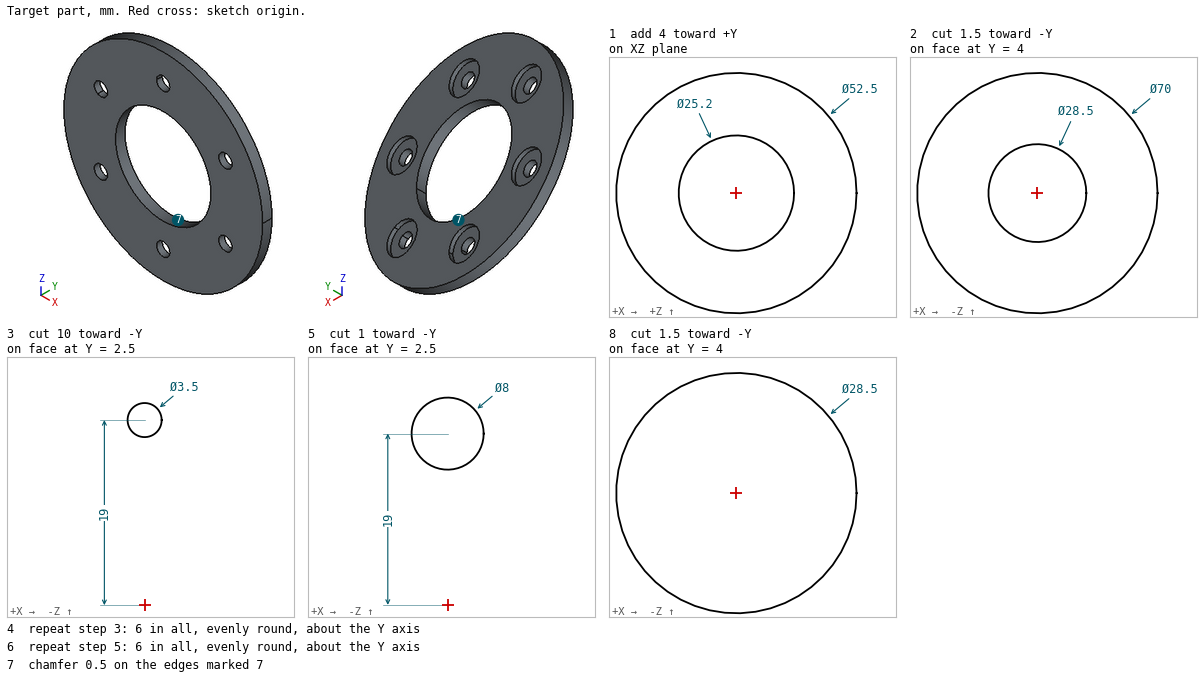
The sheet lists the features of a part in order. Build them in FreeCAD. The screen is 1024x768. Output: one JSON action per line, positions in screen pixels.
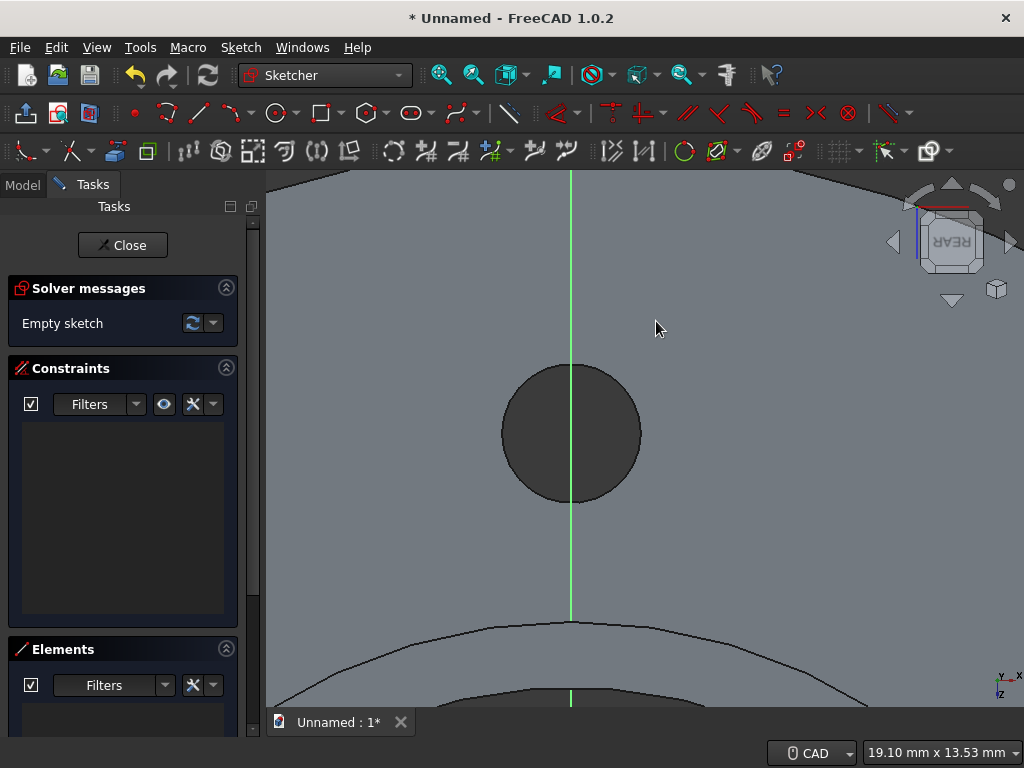
{"action": "left_click", "coordinate": [276, 114]}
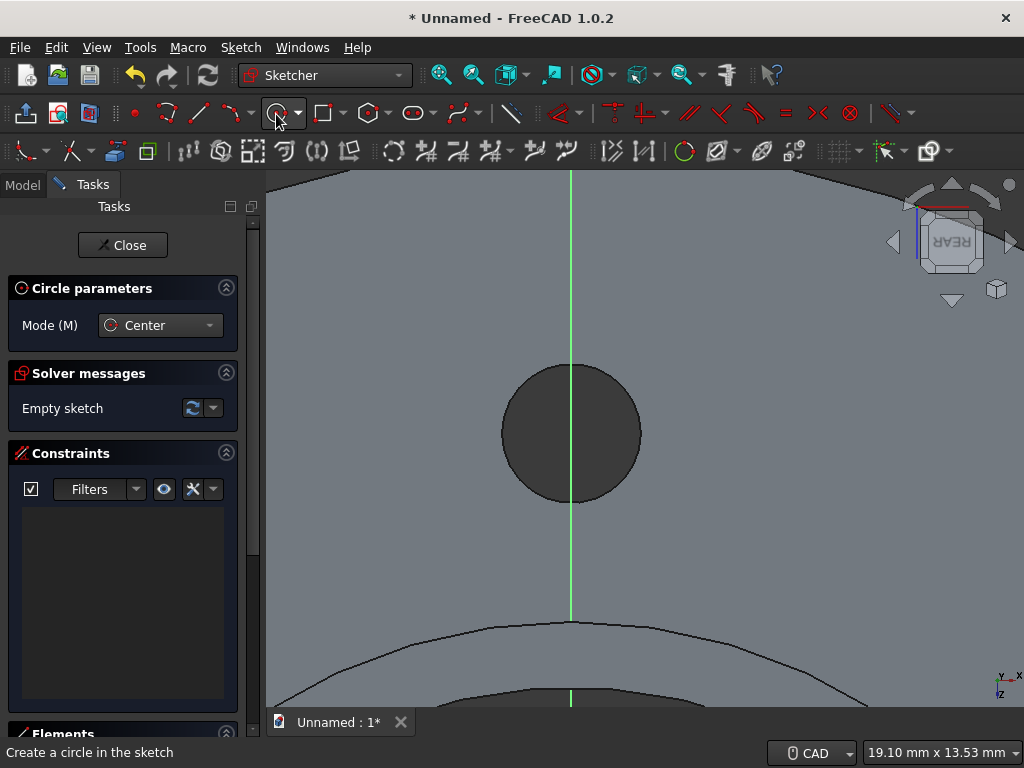
{"action": "left_click", "coordinate": [571, 434]}
{"action": "mouse_move", "coordinate": [684, 321]}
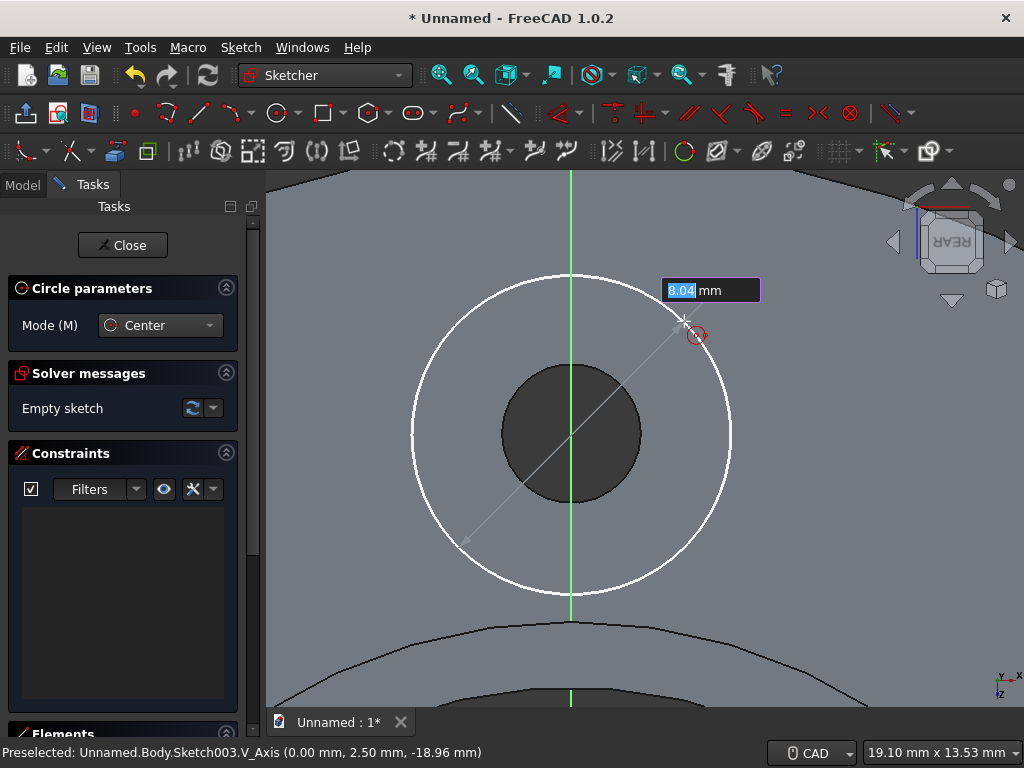
{"action": "type", "text": "8"}
{"action": "key", "text": "Return"}
{"action": "key", "text": "Escape"}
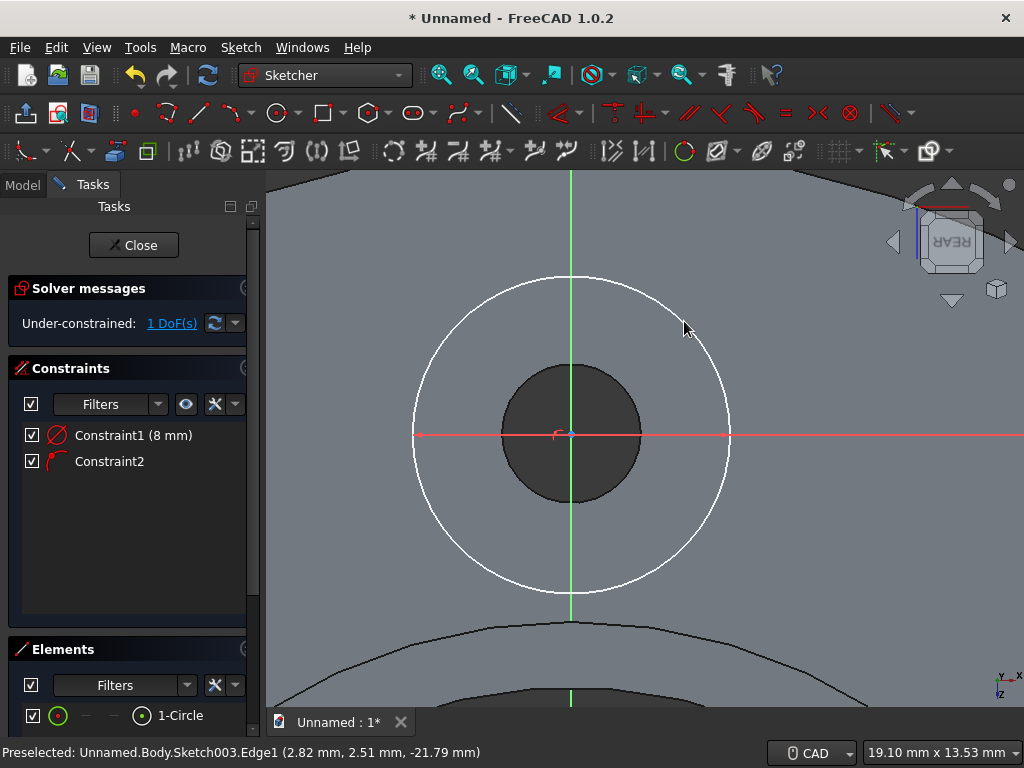
{"action": "left_click", "coordinate": [558, 114]}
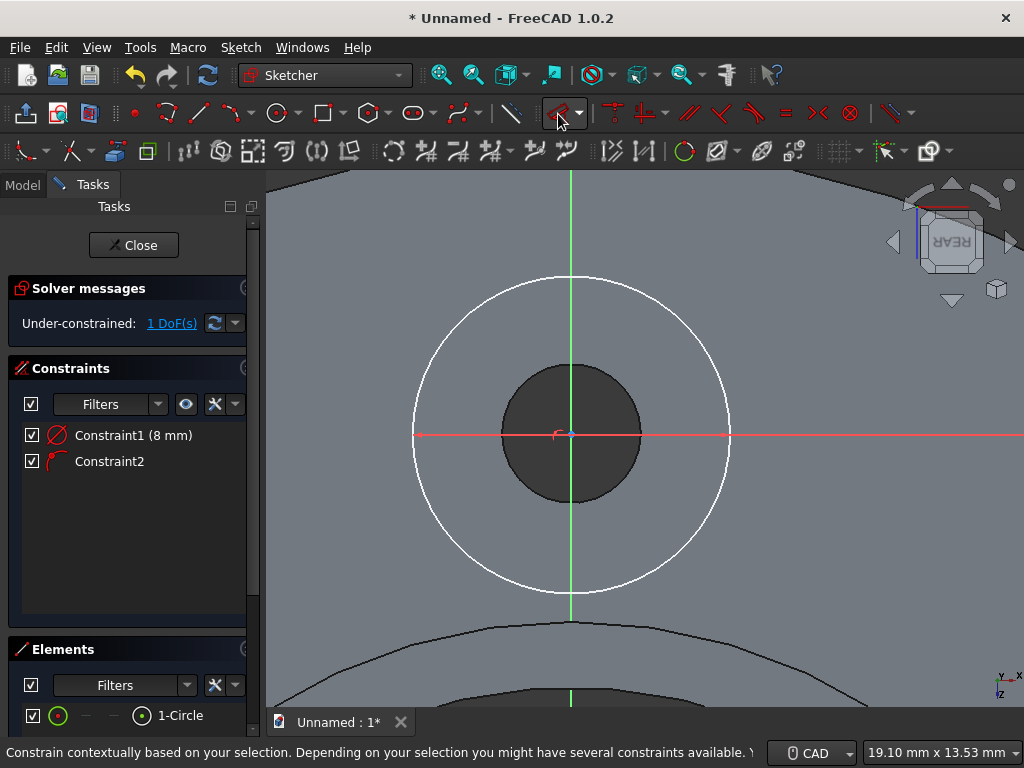
{"action": "left_click", "coordinate": [571, 435]}
{"action": "left_click", "coordinate": [605, 557]}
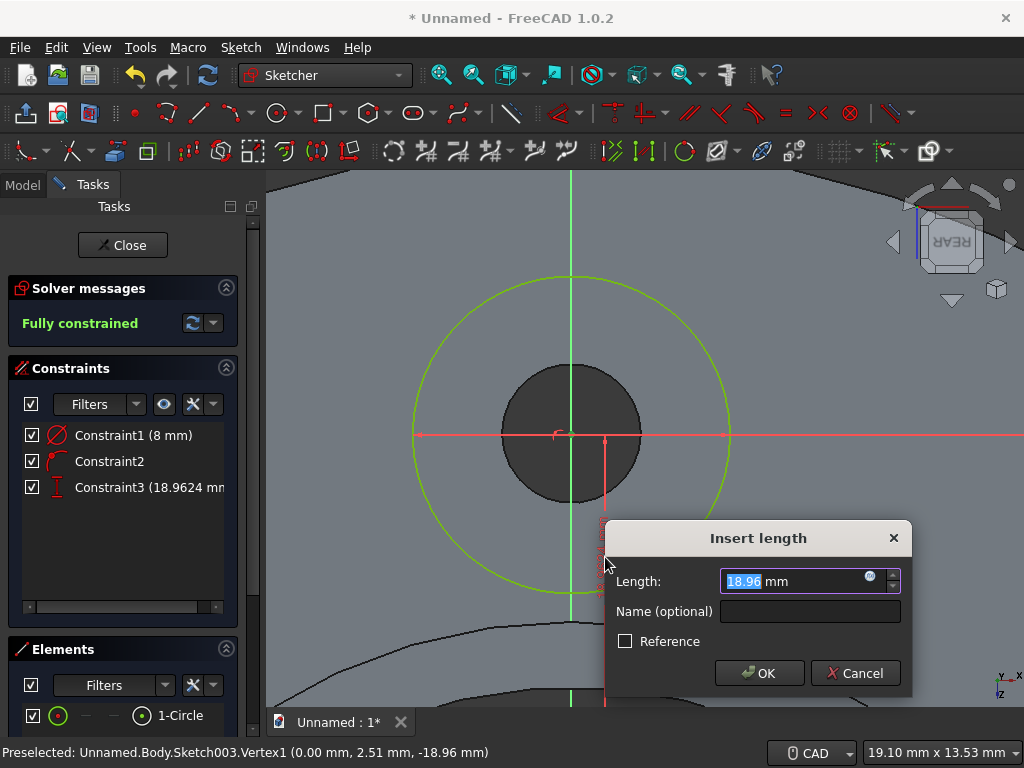
{"action": "type", "text": "19"}
{"action": "key", "text": "Return"}
{"action": "key", "text": "Escape"}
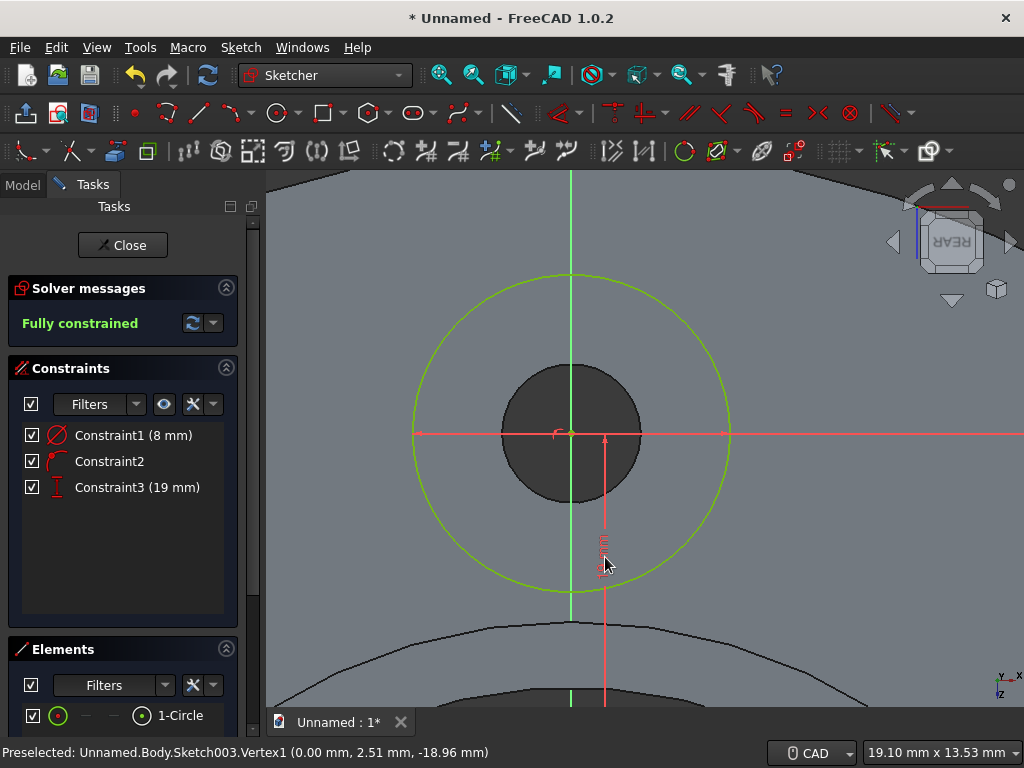
{"action": "left_click", "coordinate": [123, 245]}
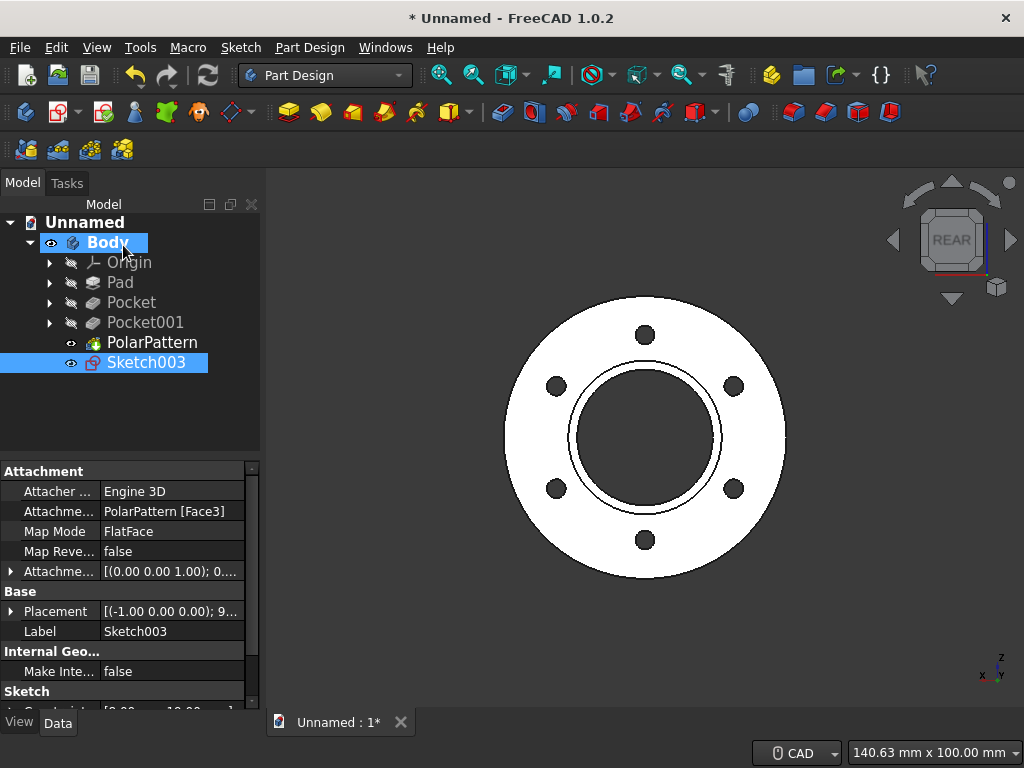
{"action": "left_click", "coordinate": [504, 112]}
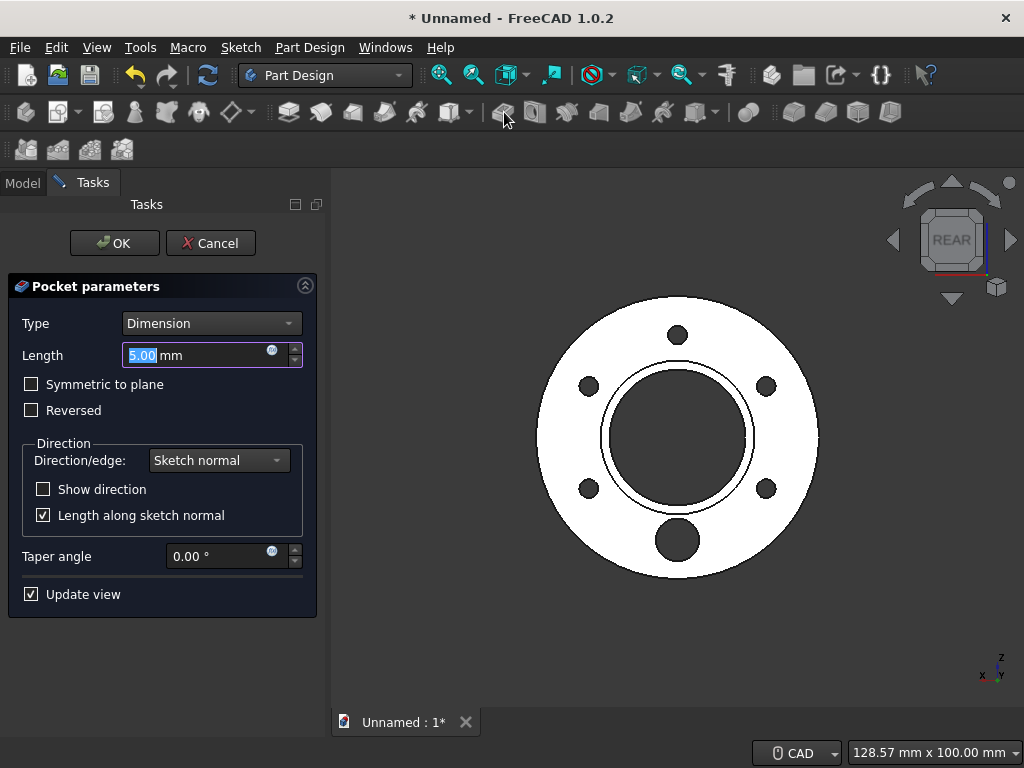
{"action": "type", "text": "1"}
{"action": "key", "text": "Tab"}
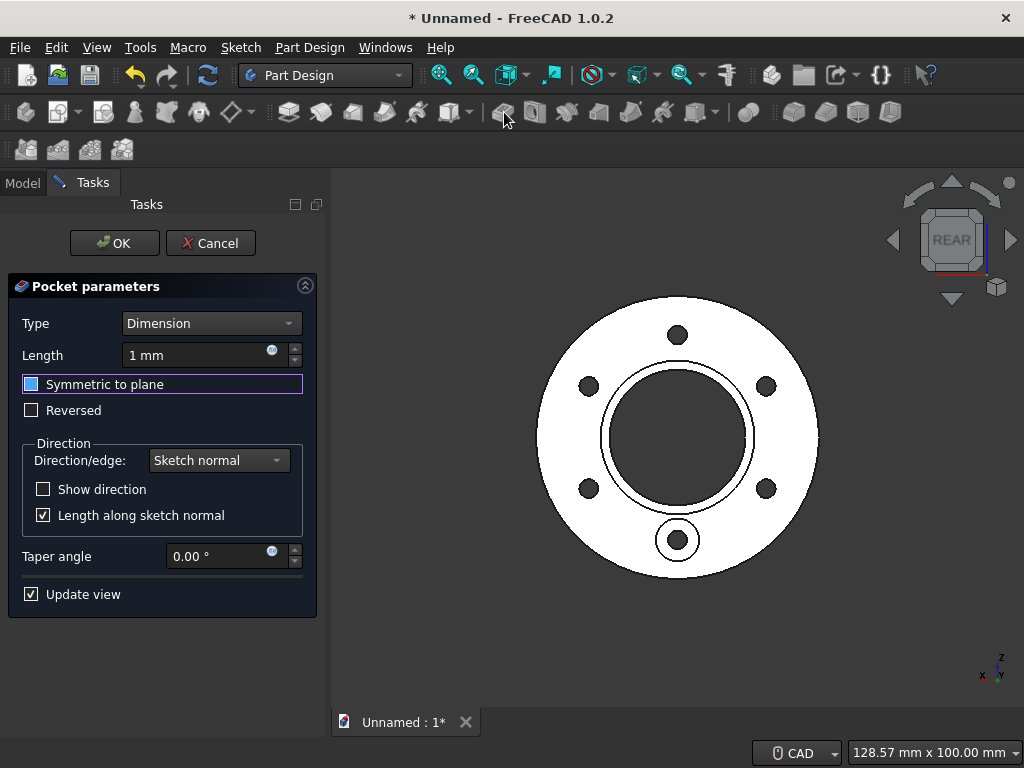
{"action": "left_click", "coordinate": [115, 243]}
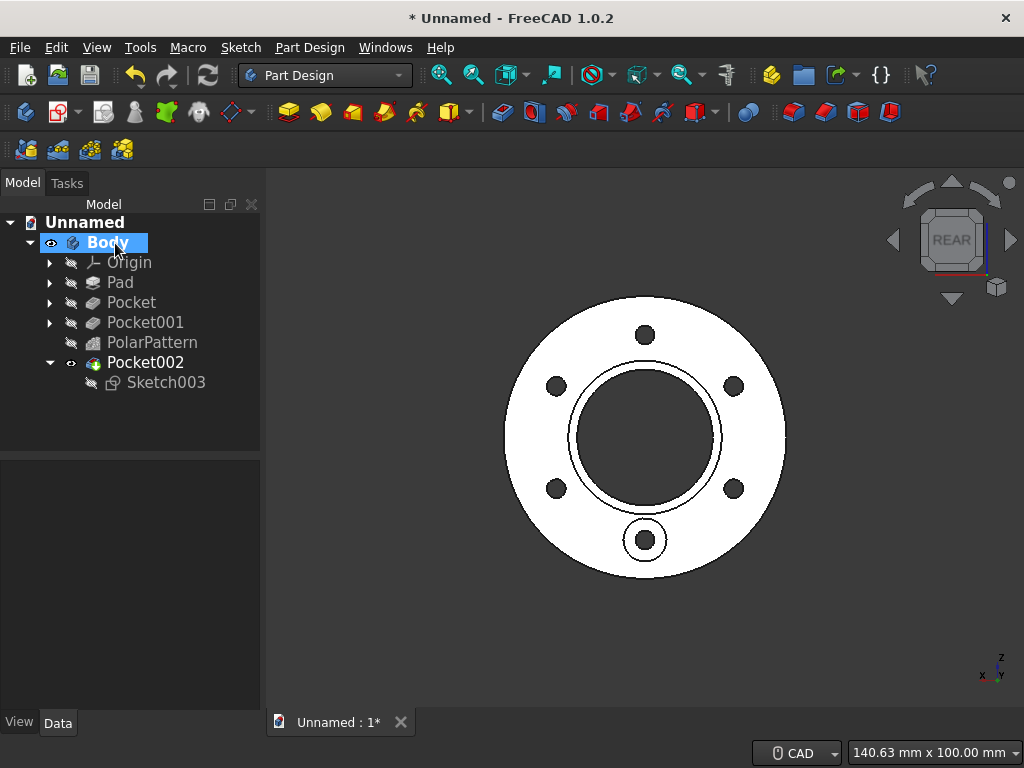
{"action": "left_click", "coordinate": [116, 363]}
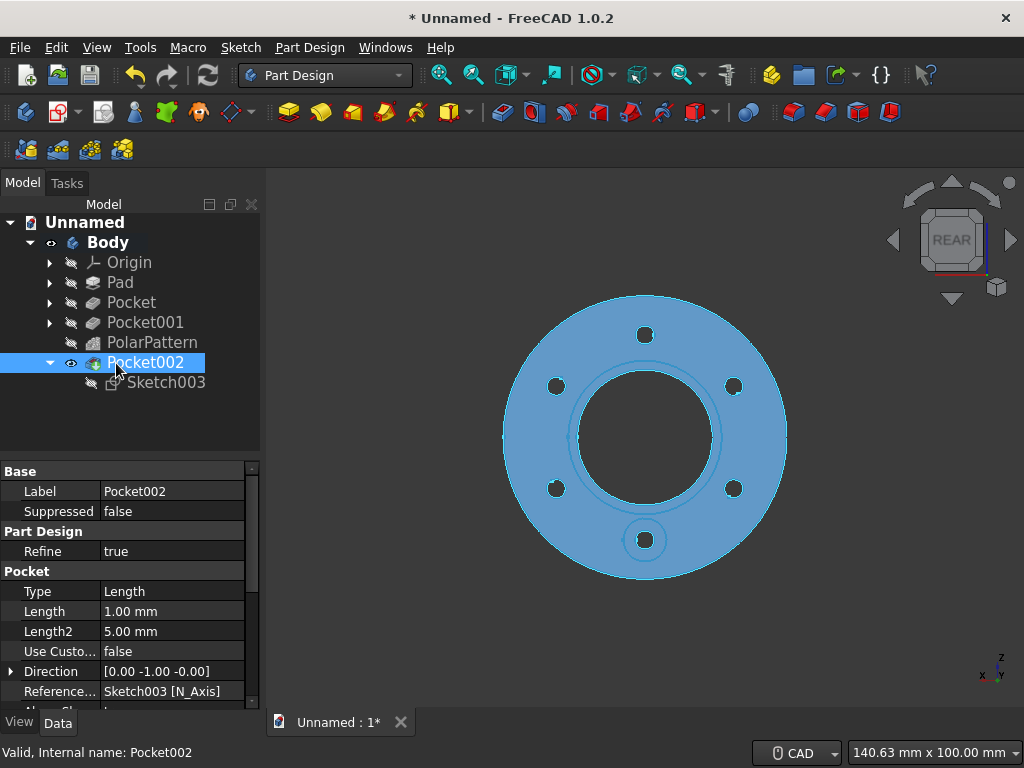
{"action": "left_click", "coordinate": [90, 150]}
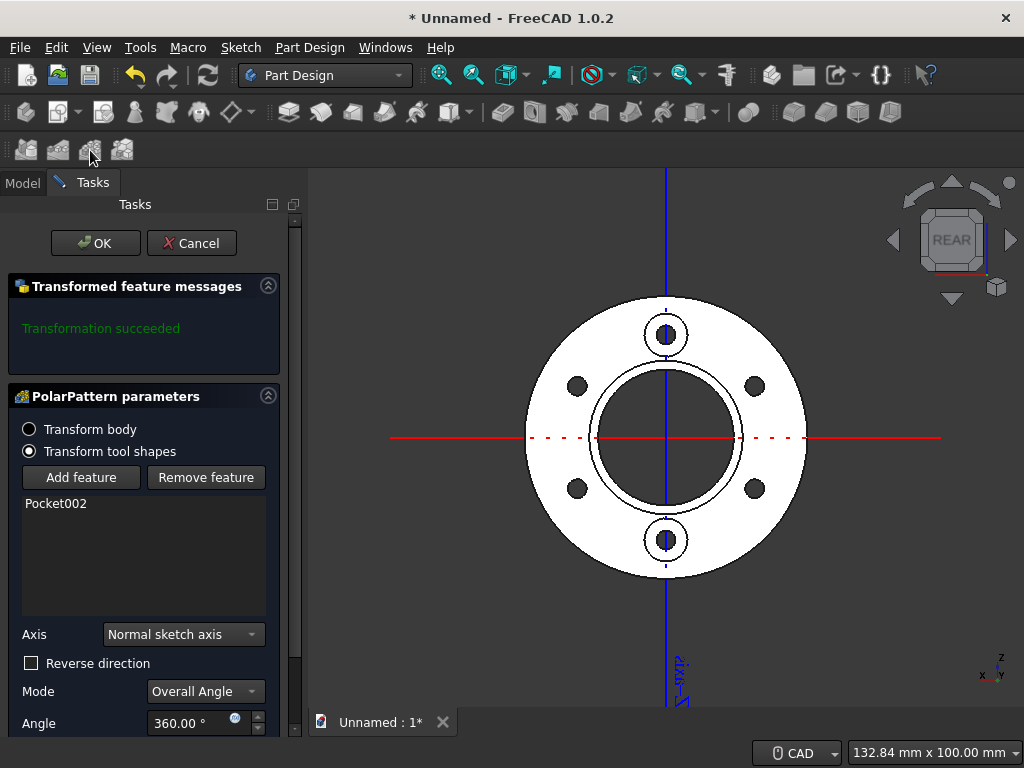
{"action": "left_click", "coordinate": [184, 634]}